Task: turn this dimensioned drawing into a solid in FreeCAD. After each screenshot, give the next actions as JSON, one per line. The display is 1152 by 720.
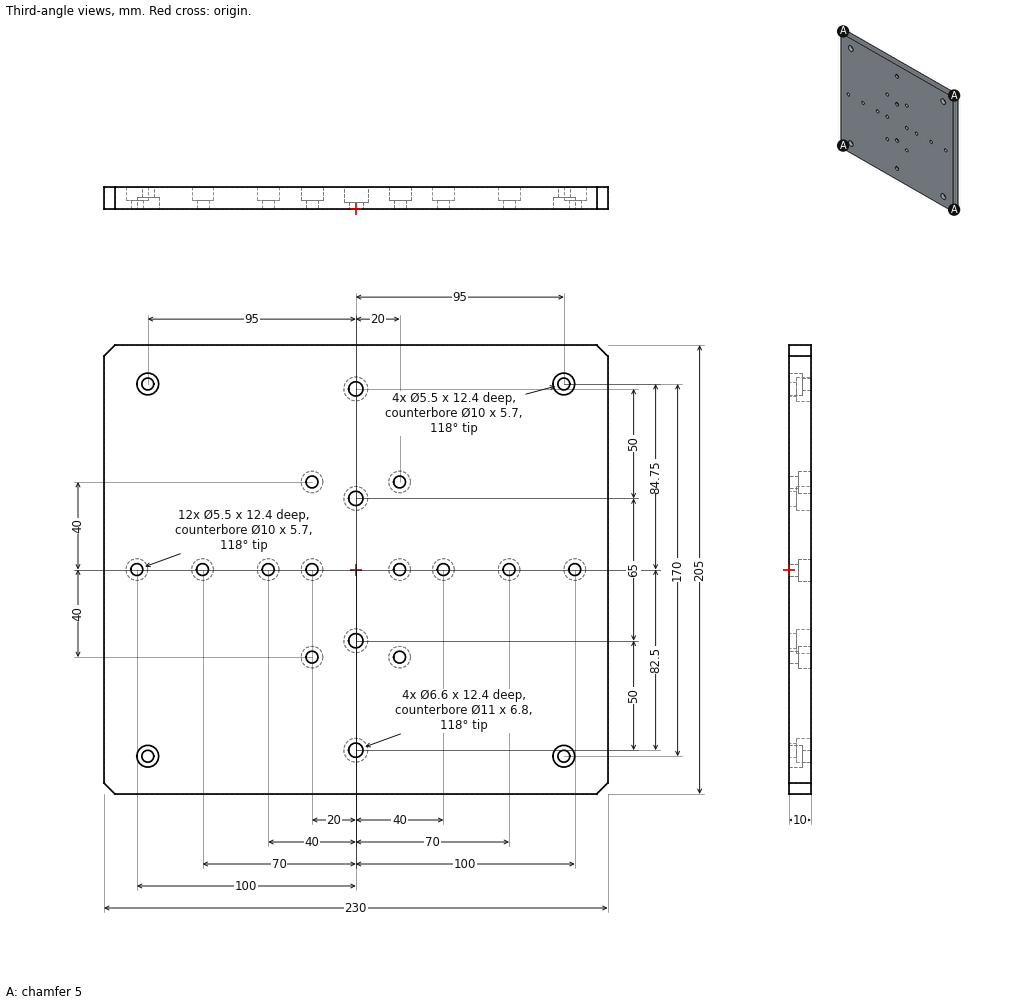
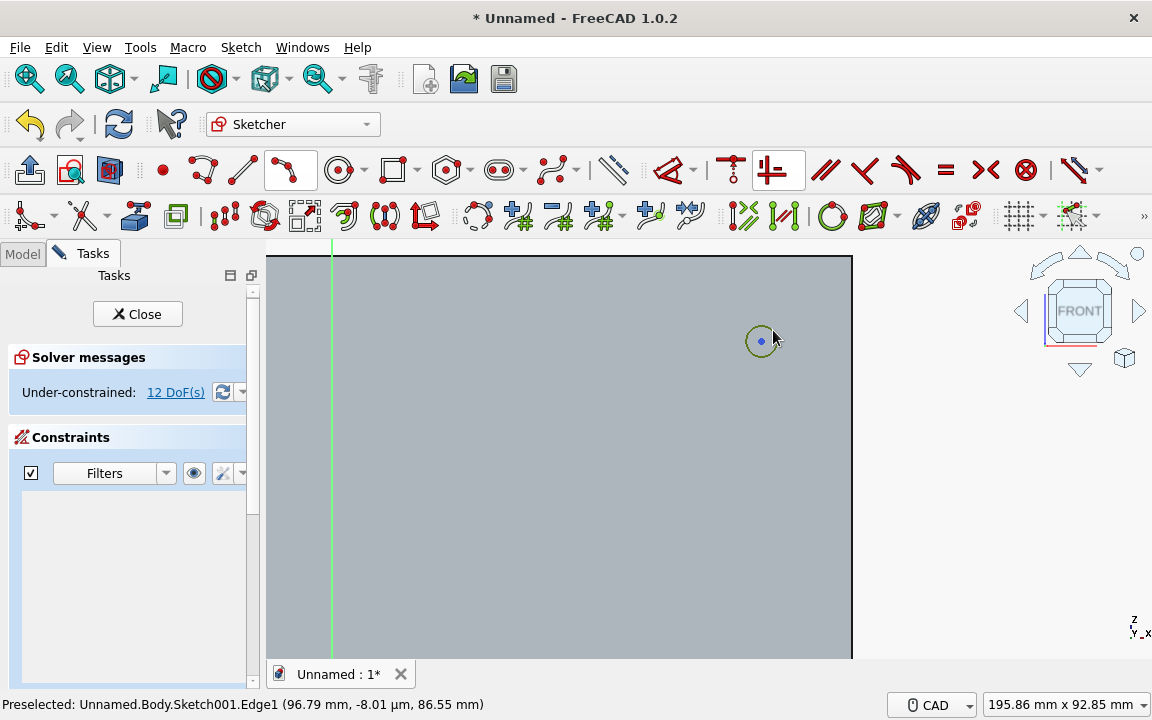
{"action": "scroll", "coordinate": [773, 332], "scroll_direction": "down", "scroll_amount": 6}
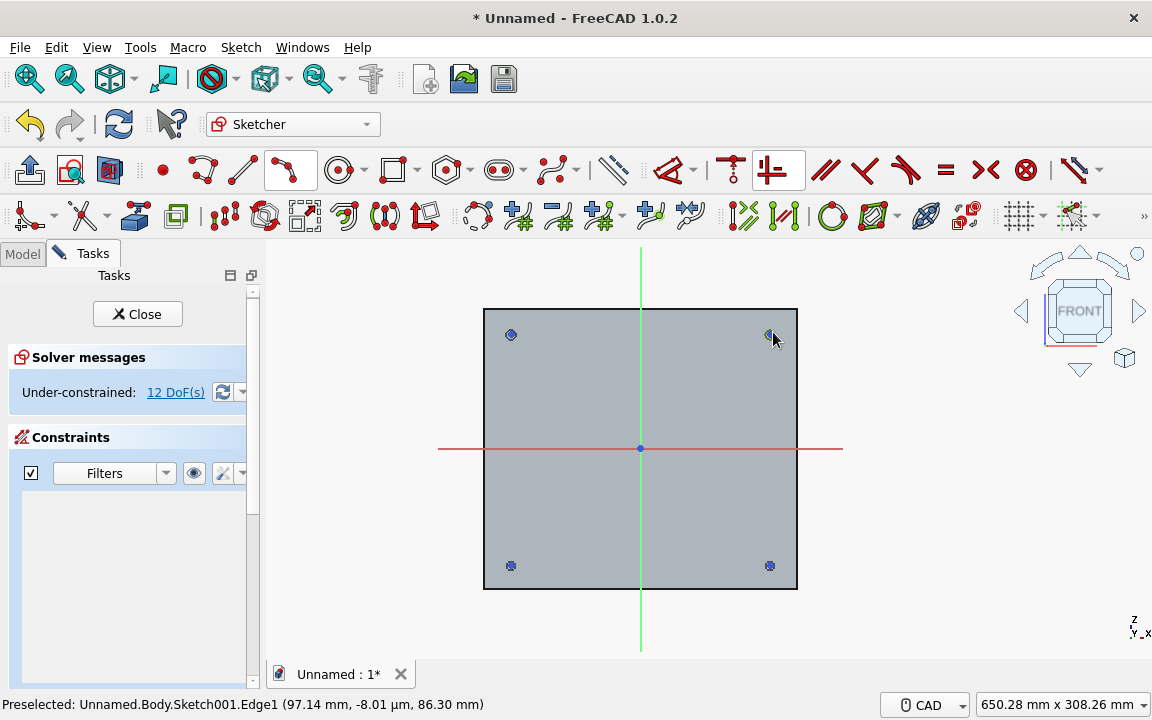
{"action": "scroll", "coordinate": [773, 563], "scroll_direction": "up", "scroll_amount": 6}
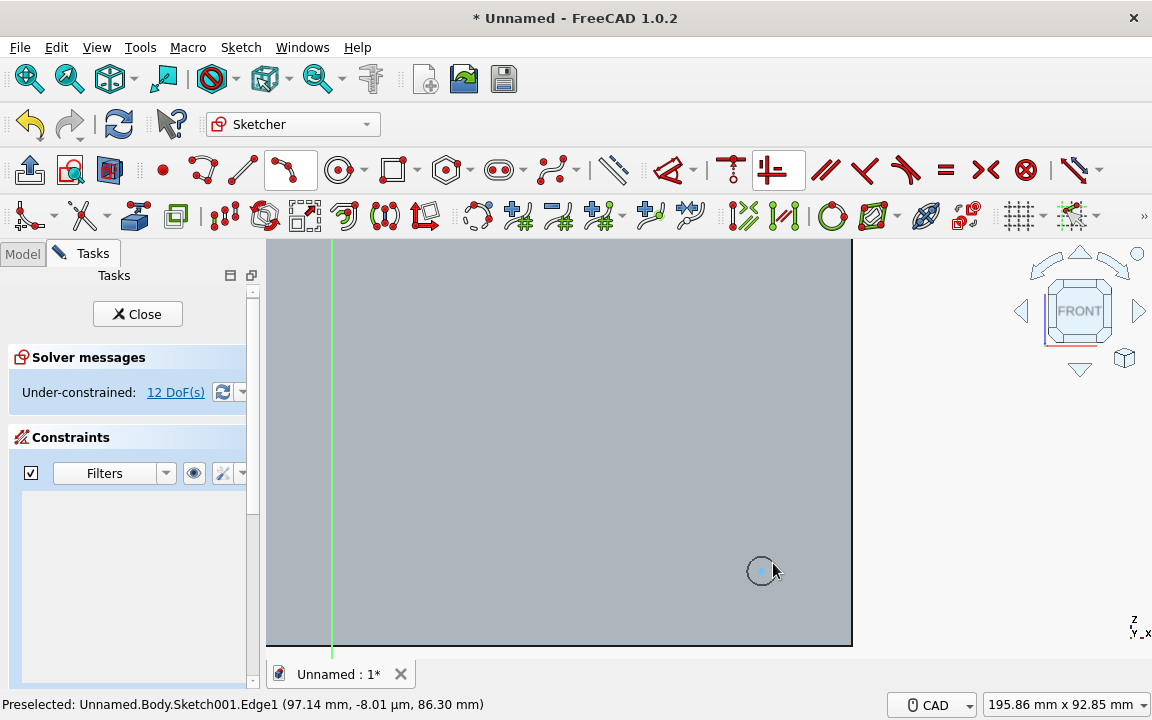
{"action": "left_click", "coordinate": [772, 561]}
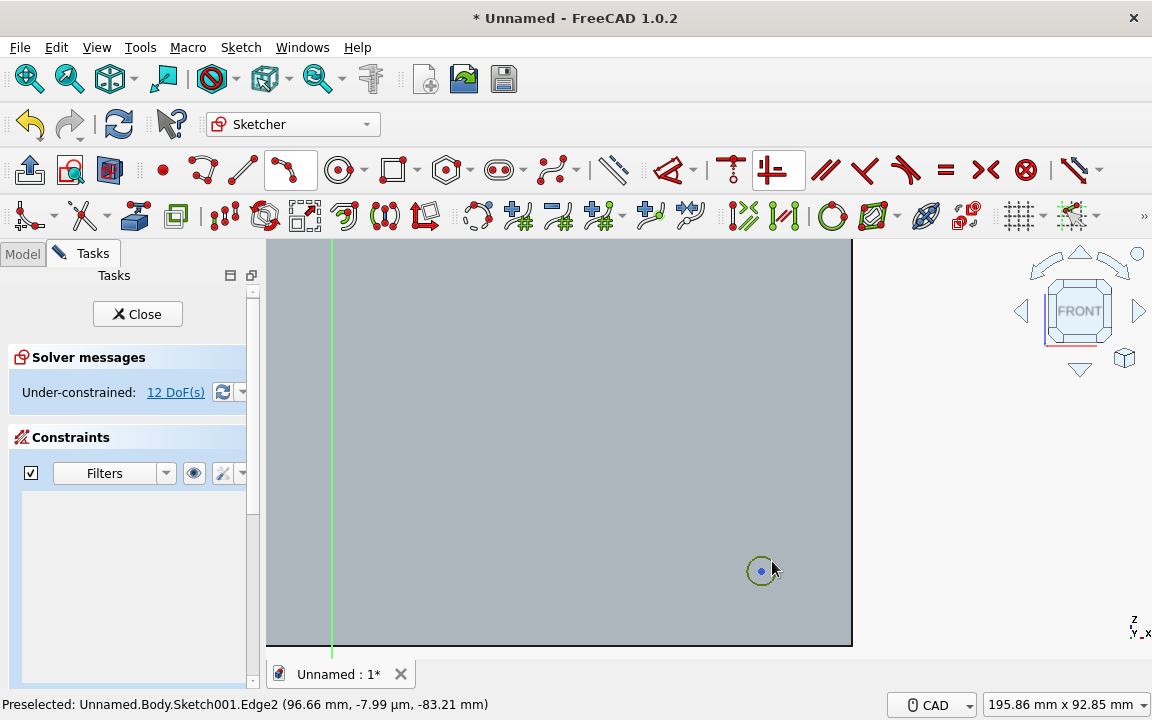
{"action": "scroll", "coordinate": [773, 563], "scroll_direction": "down", "scroll_amount": 6}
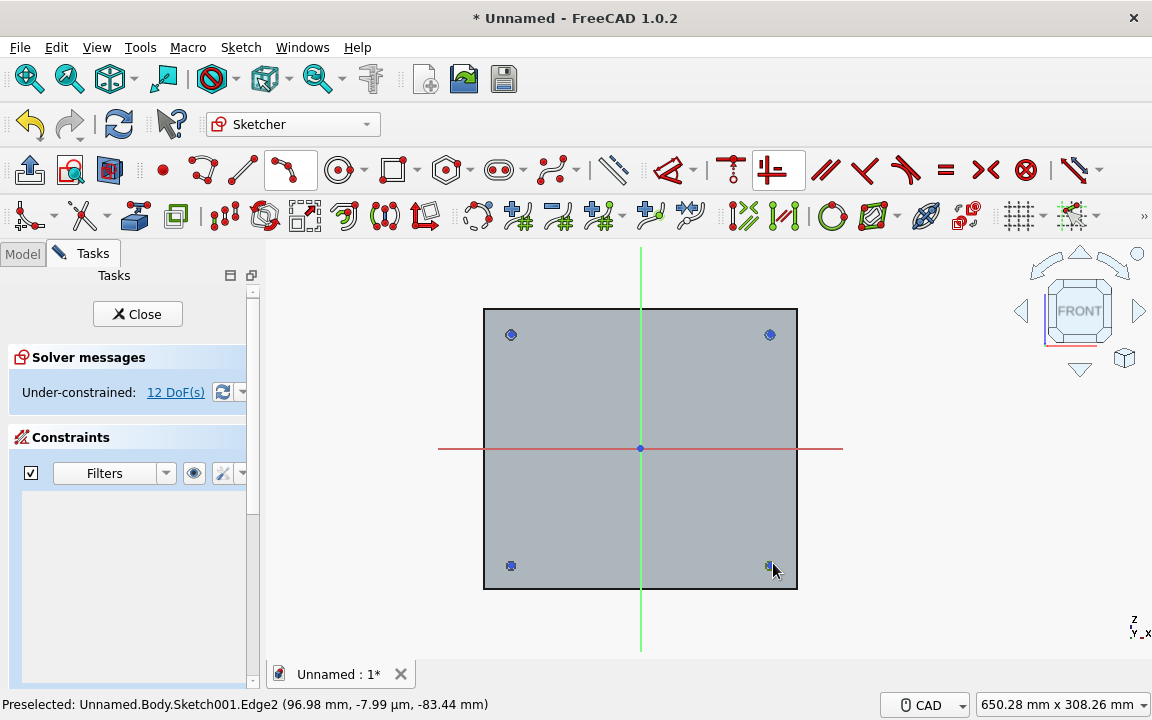
{"action": "scroll", "coordinate": [514, 332], "scroll_direction": "up", "scroll_amount": 6}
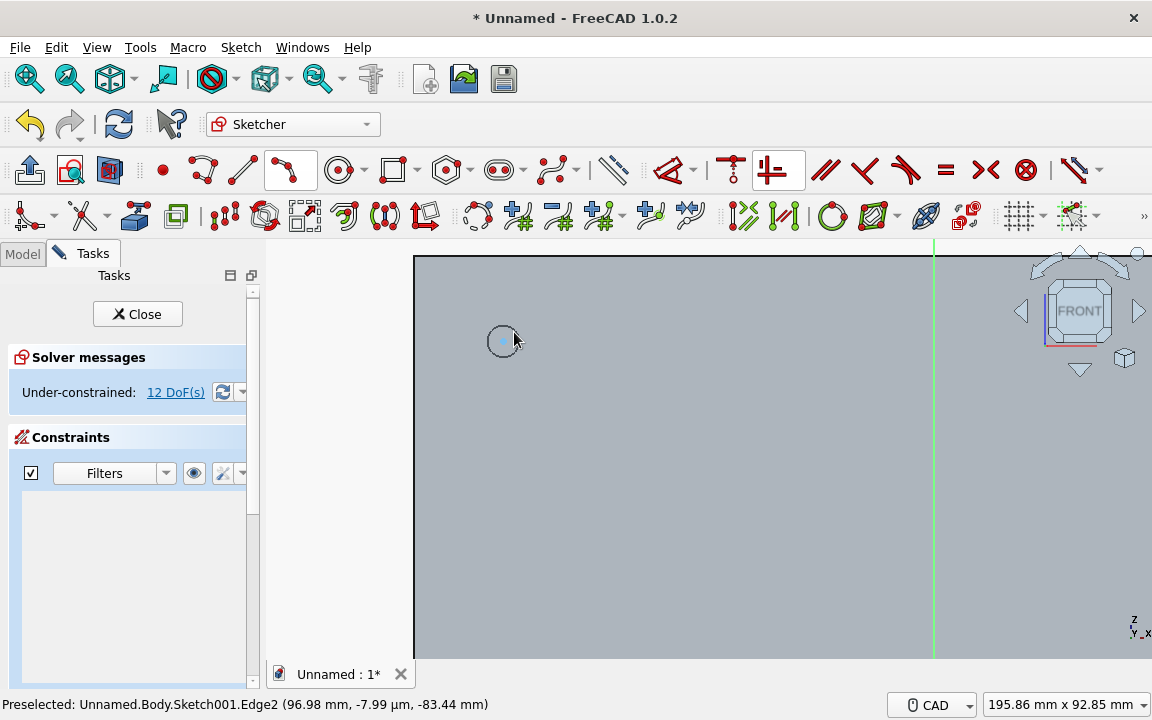
{"action": "left_click", "coordinate": [515, 330]}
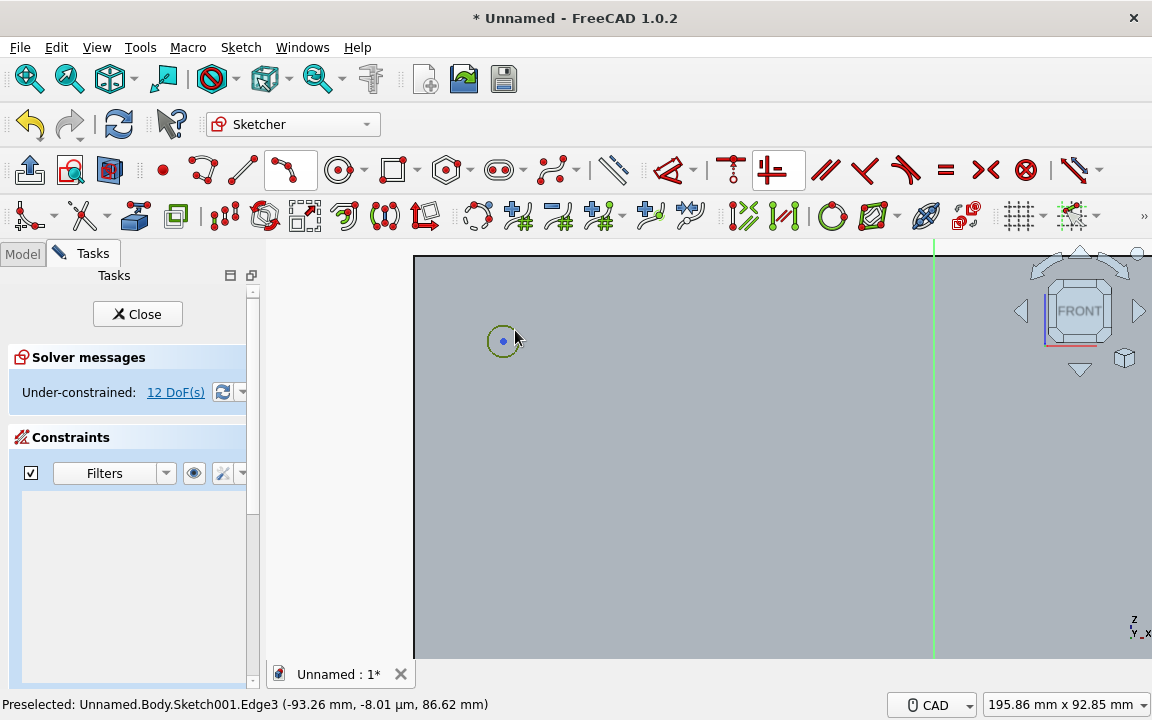
{"action": "scroll", "coordinate": [514, 332], "scroll_direction": "down", "scroll_amount": 6}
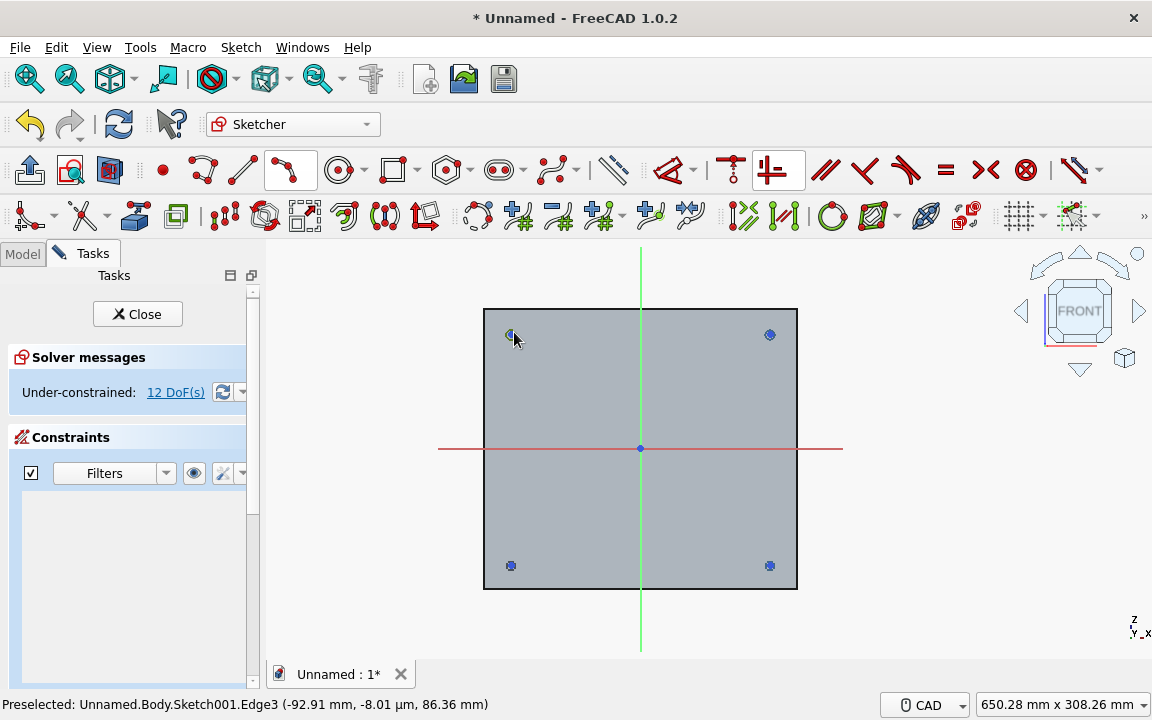
{"action": "scroll", "coordinate": [514, 563], "scroll_direction": "up", "scroll_amount": 6}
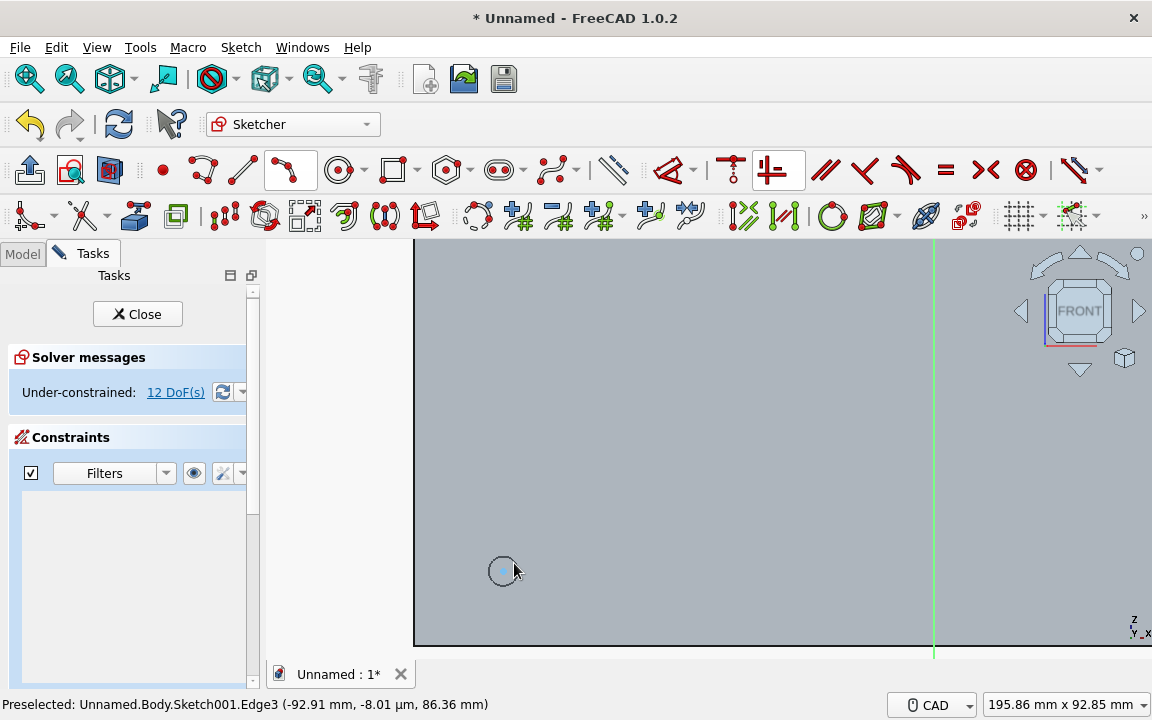
{"action": "left_click", "coordinate": [514, 561]}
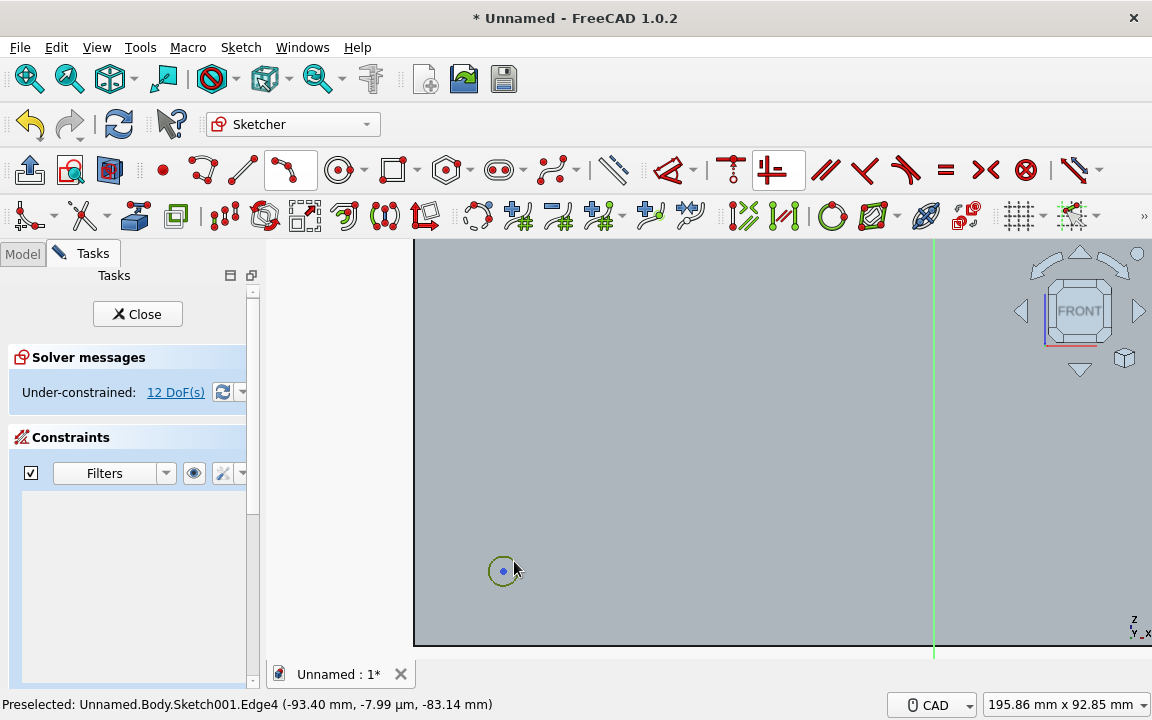
{"action": "left_click", "coordinate": [946, 170]}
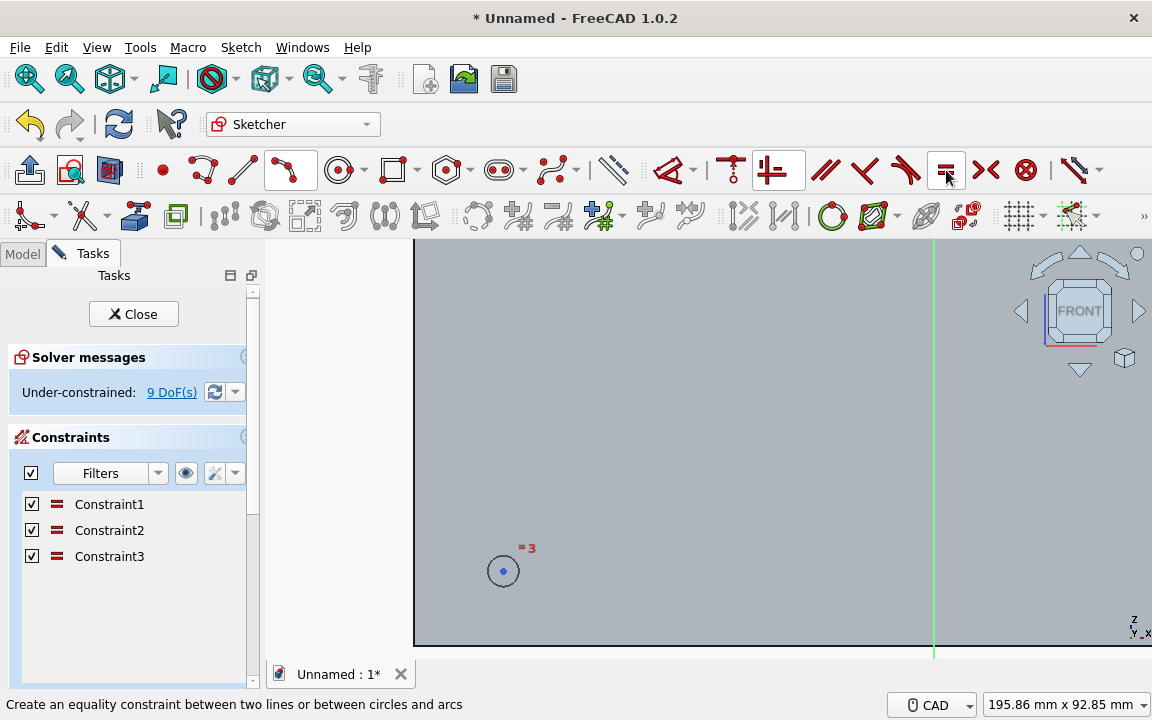
{"action": "scroll", "coordinate": [514, 563], "scroll_direction": "down", "scroll_amount": 6}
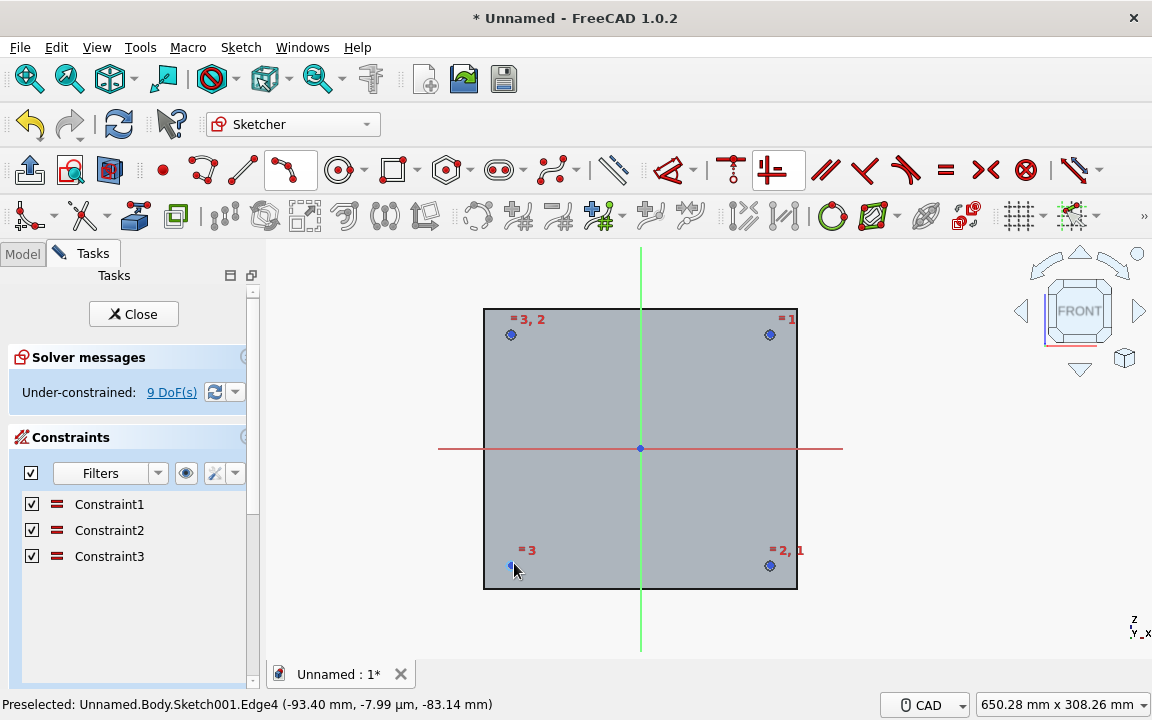
{"action": "left_click", "coordinate": [770, 335]}